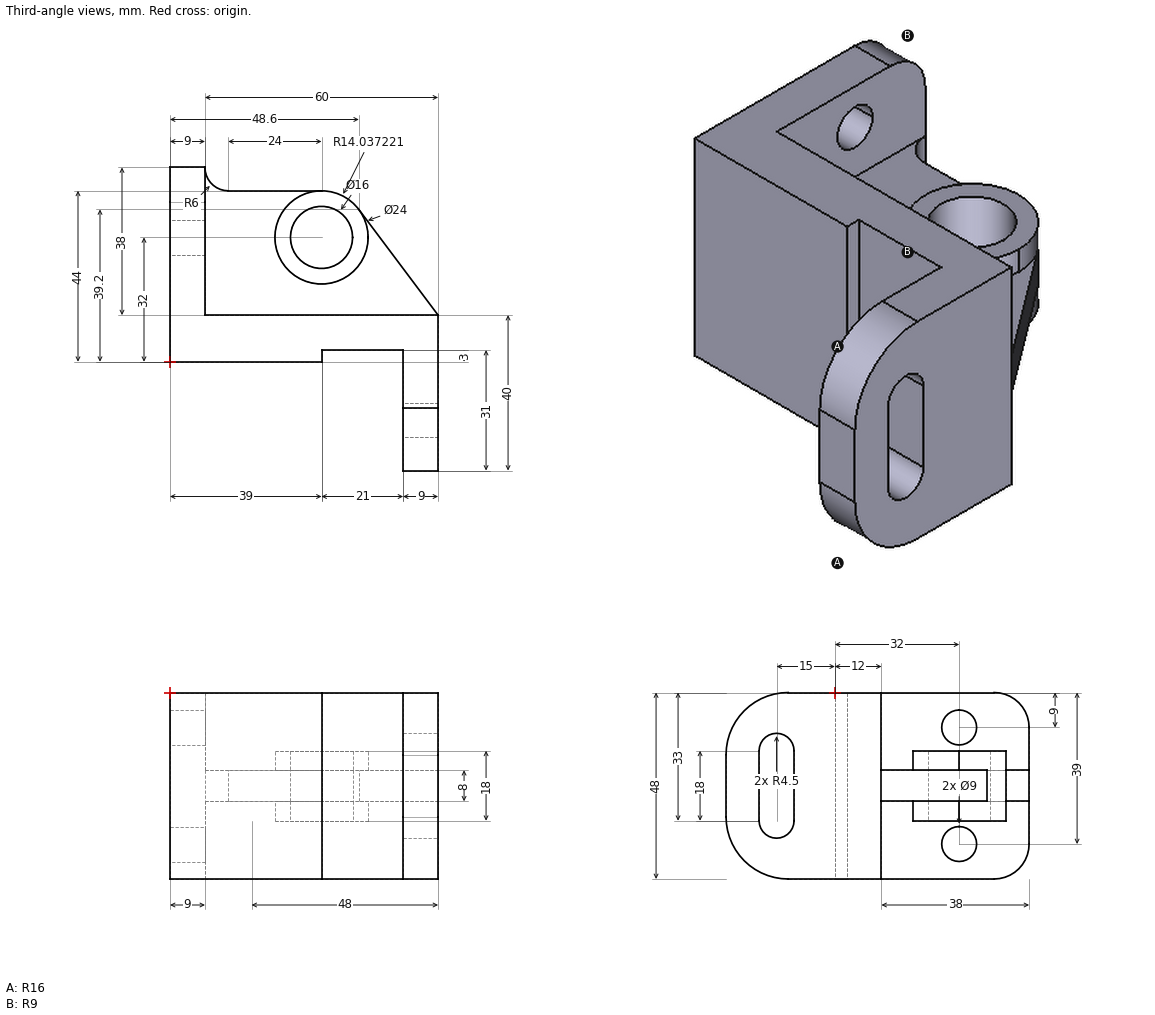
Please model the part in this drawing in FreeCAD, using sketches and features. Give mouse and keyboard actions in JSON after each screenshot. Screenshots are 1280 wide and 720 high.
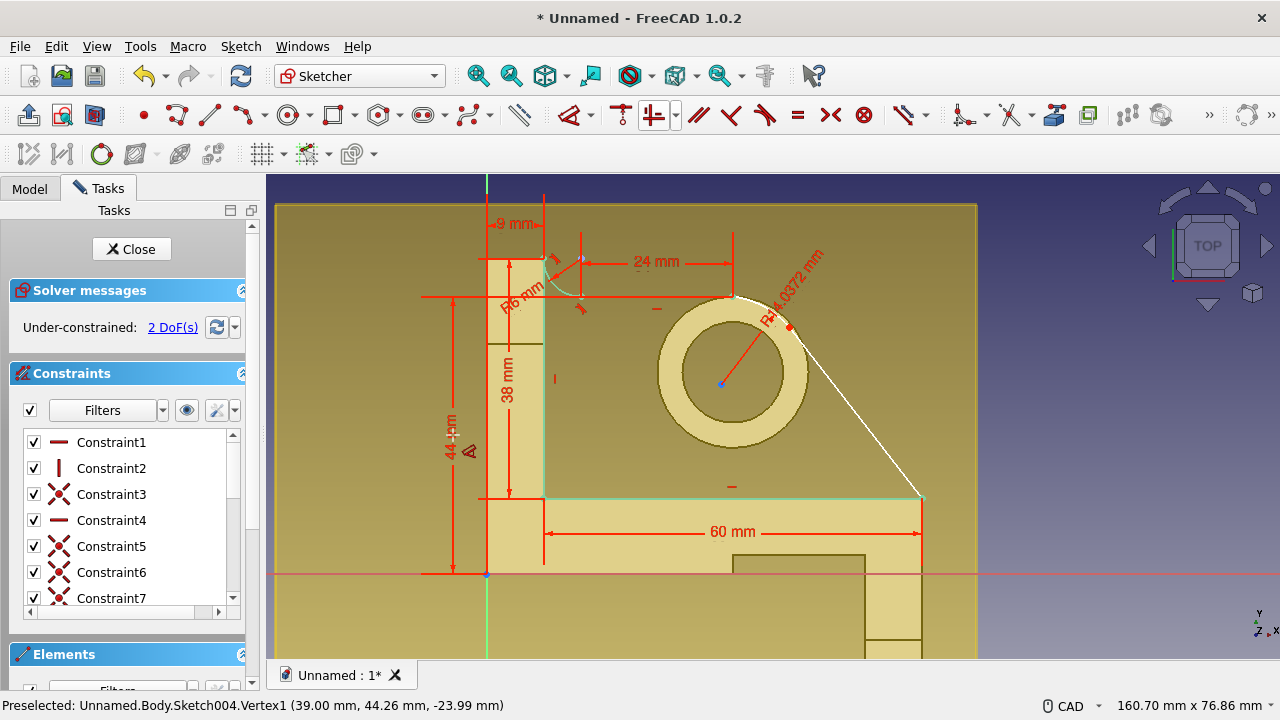
{"action": "left_click", "coordinate": [790, 328]}
{"action": "left_click", "coordinate": [638, 608]}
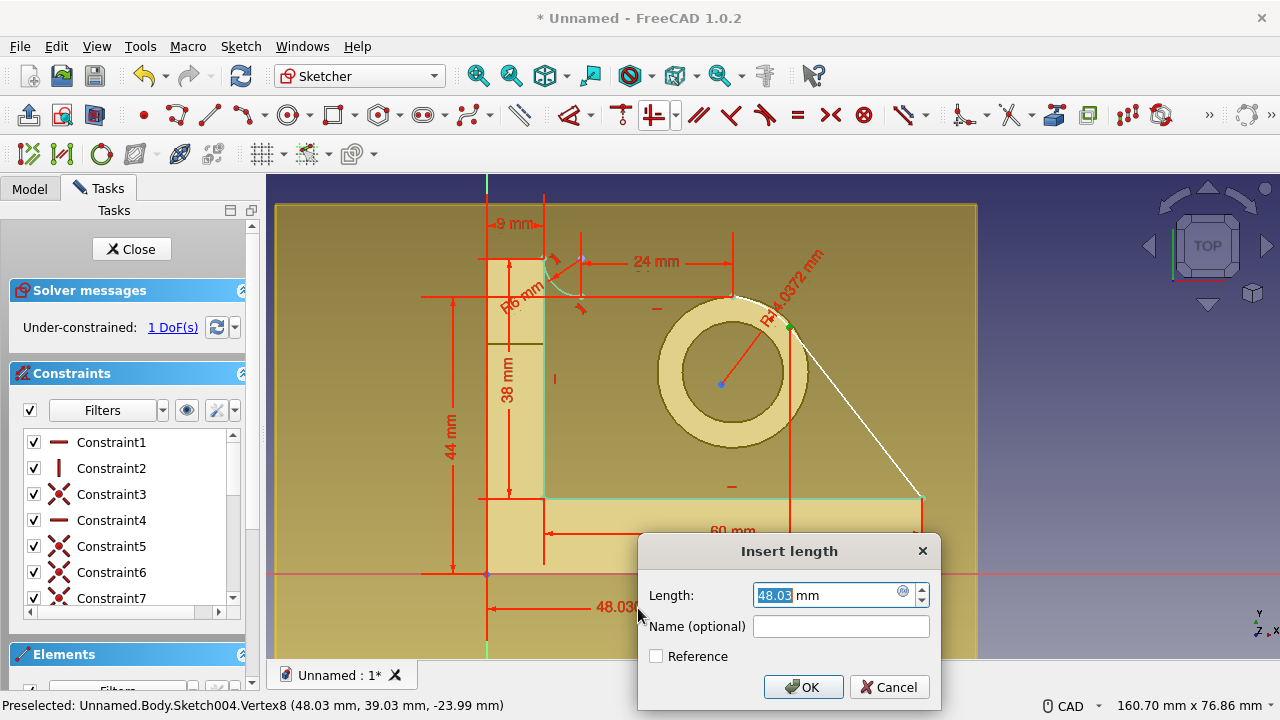
{"action": "type", "text": "48.6"}
{"action": "key", "text": "Return"}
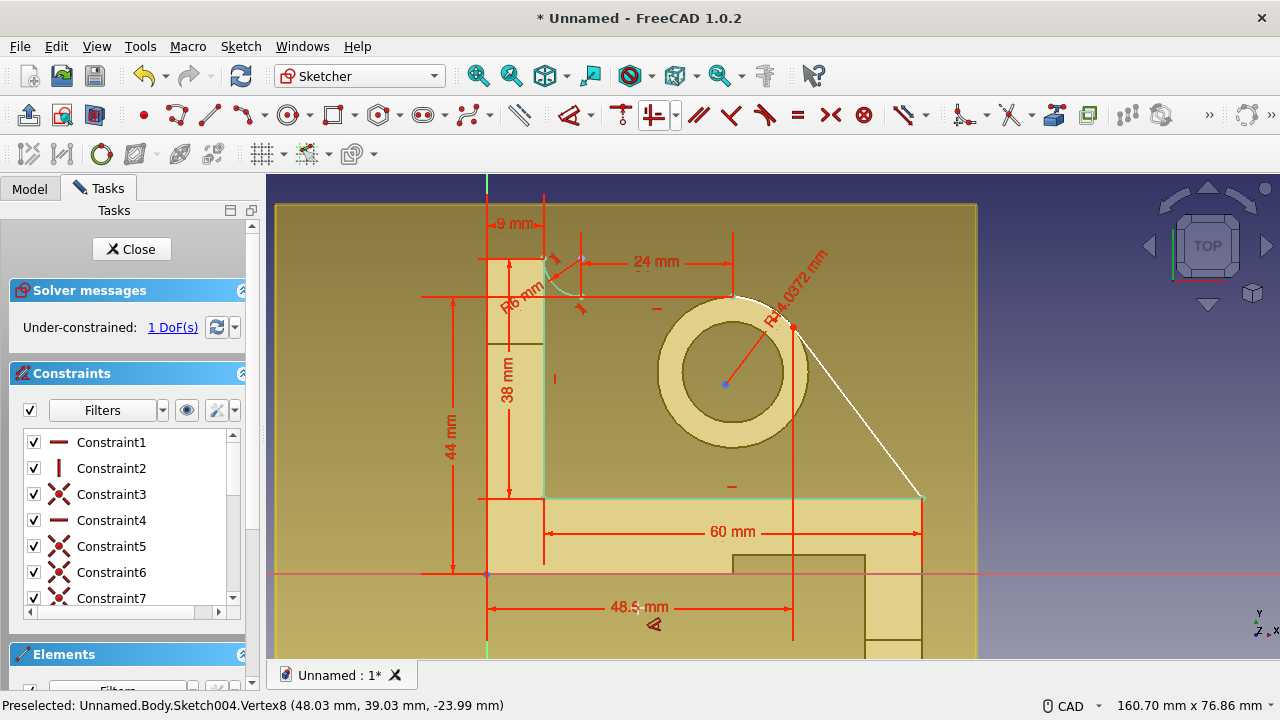
{"action": "left_click", "coordinate": [793, 328]}
{"action": "left_click", "coordinate": [453, 508]}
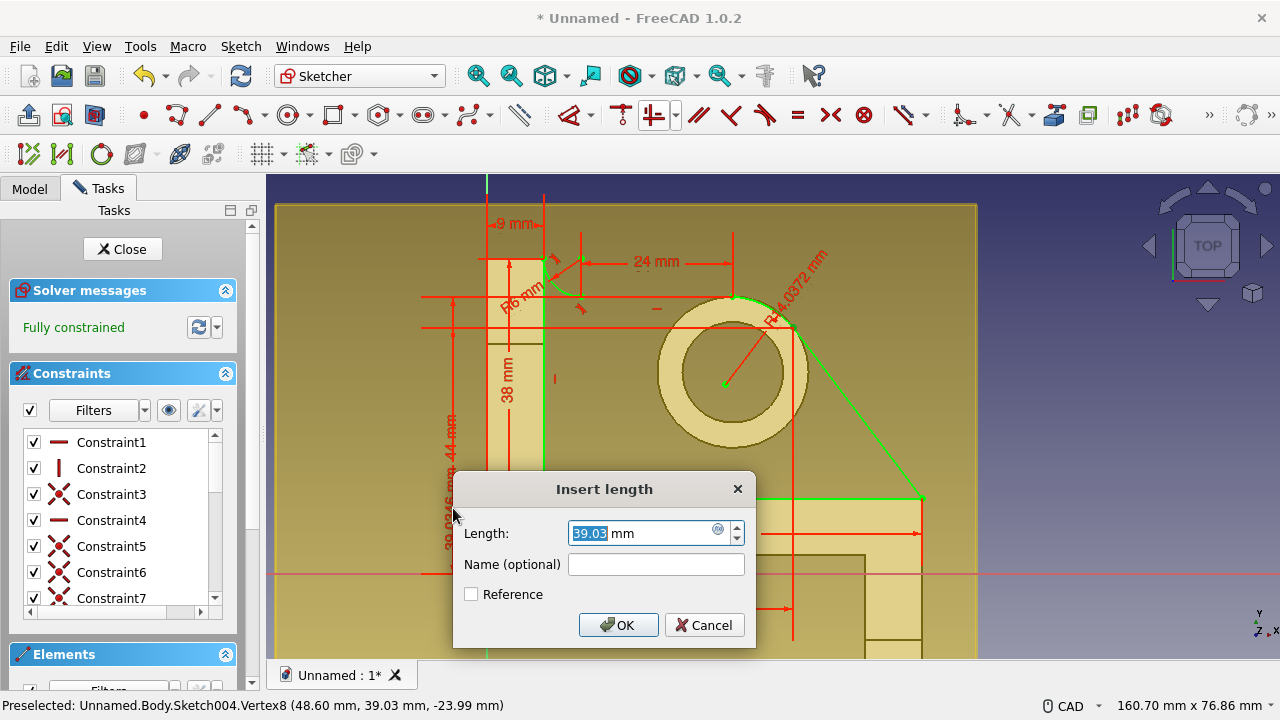
{"action": "type", "text": "39.2"}
{"action": "key", "text": "Return"}
{"action": "key", "text": "Escape"}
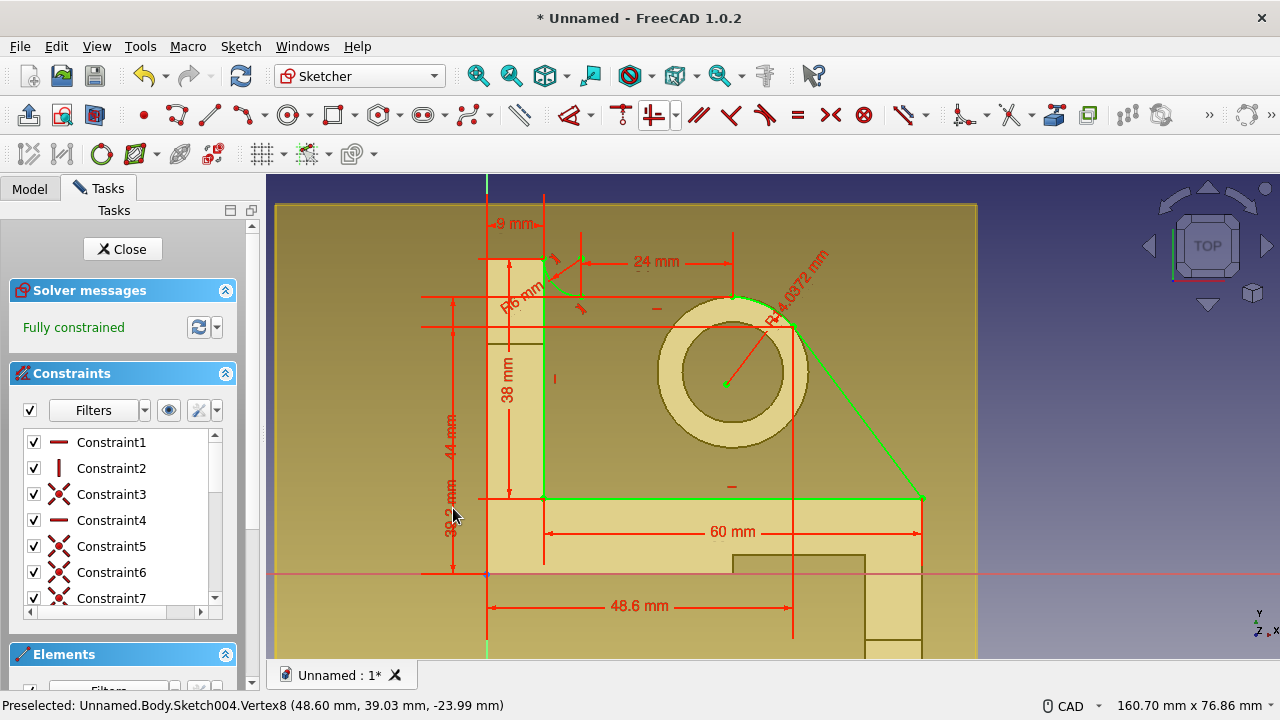
{"action": "left_click", "coordinate": [123, 249]}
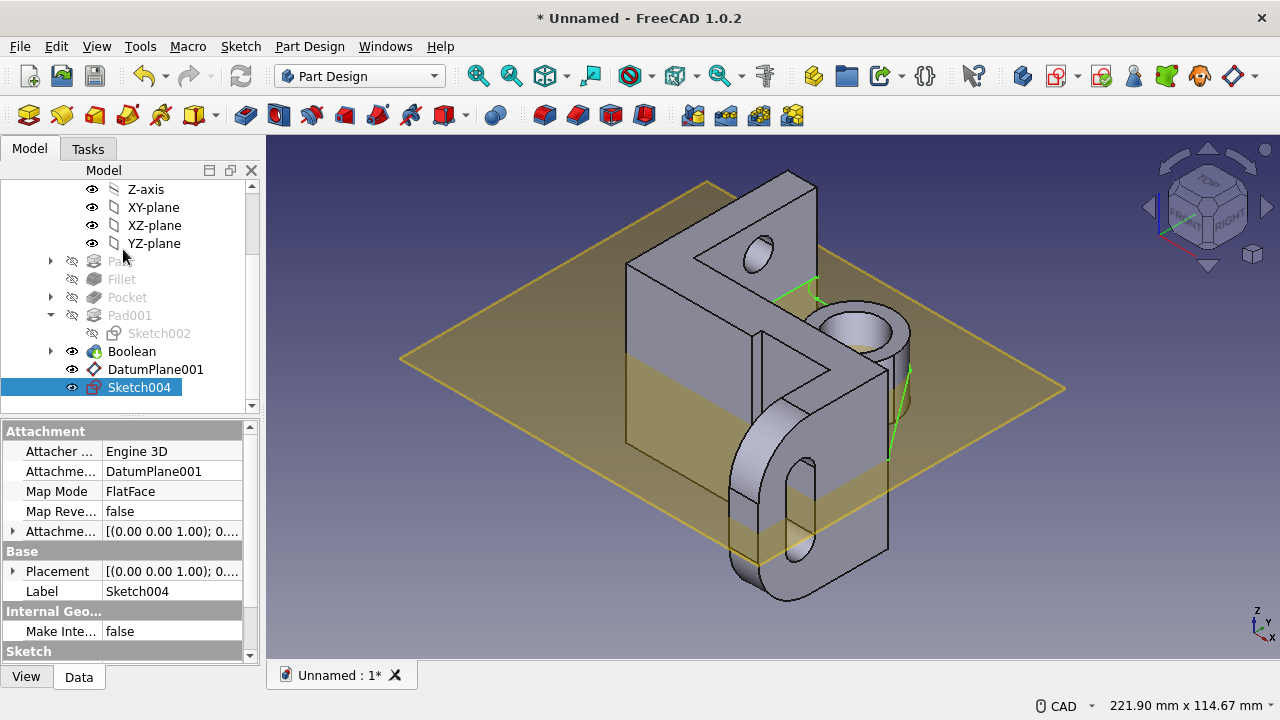
{"action": "left_click", "coordinate": [29, 116]}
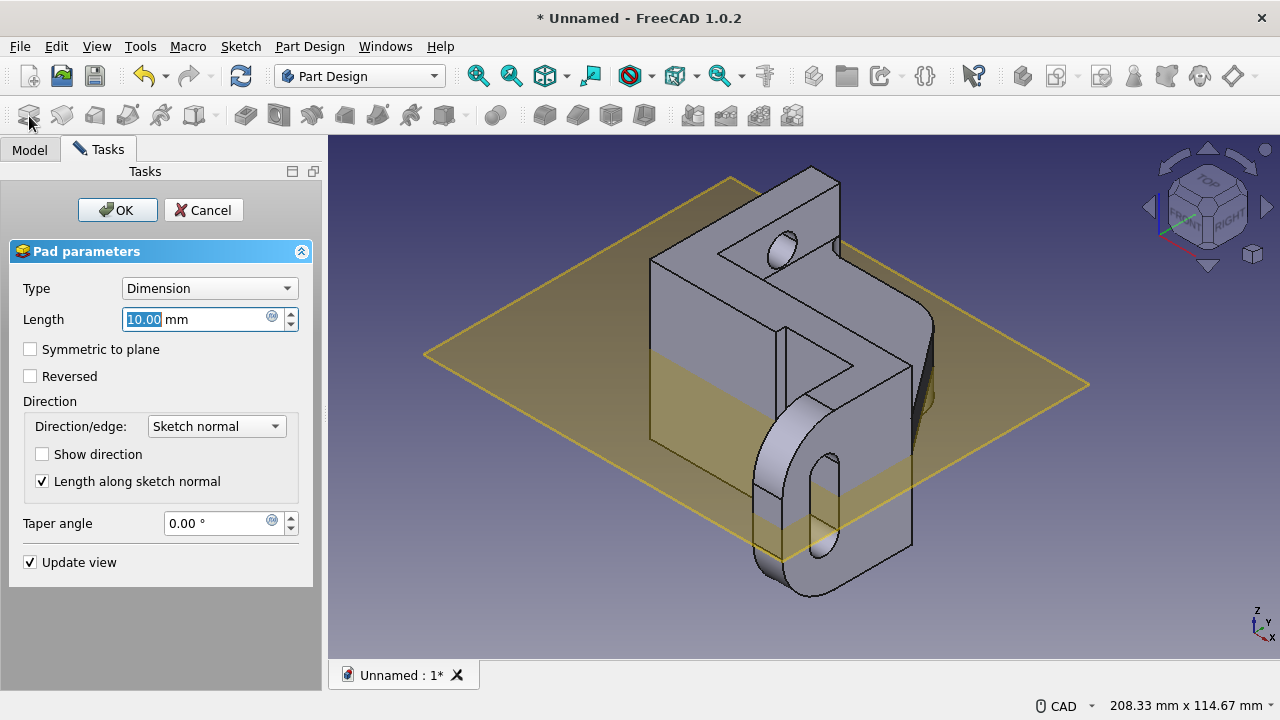
{"action": "type", "text": "8"}
{"action": "key", "text": "Tab"}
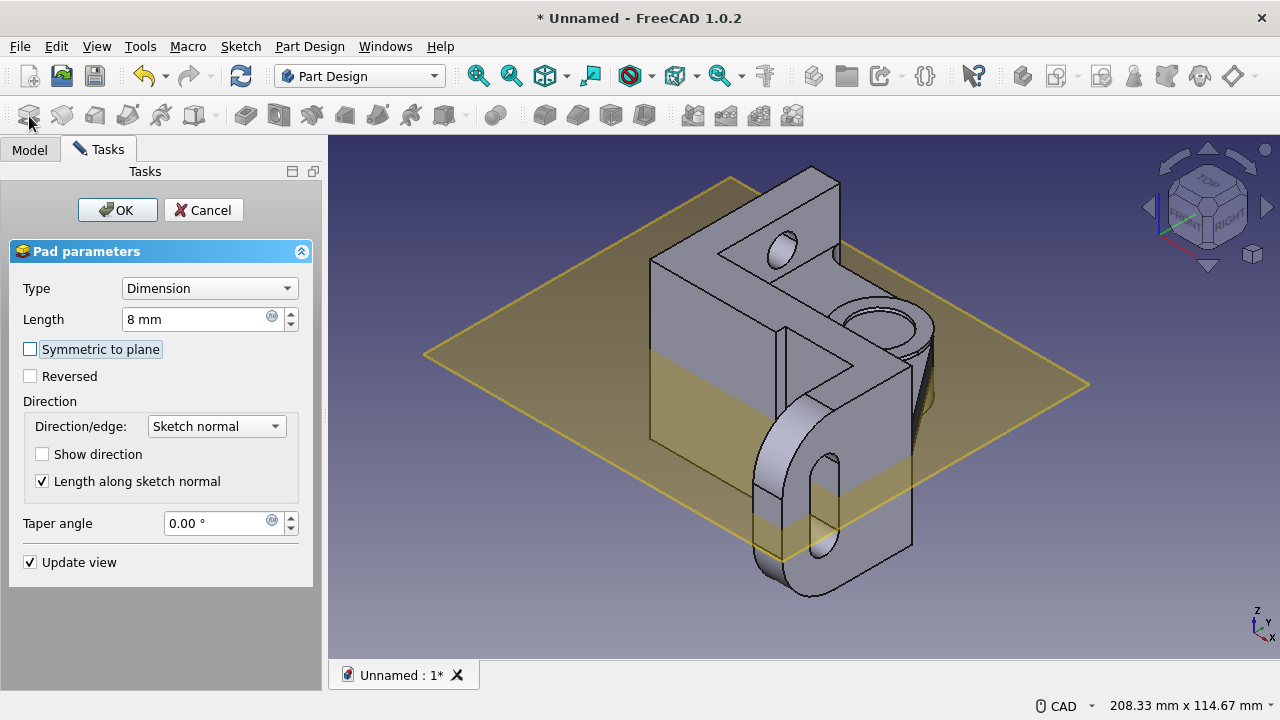
{"action": "left_click", "coordinate": [31, 349]}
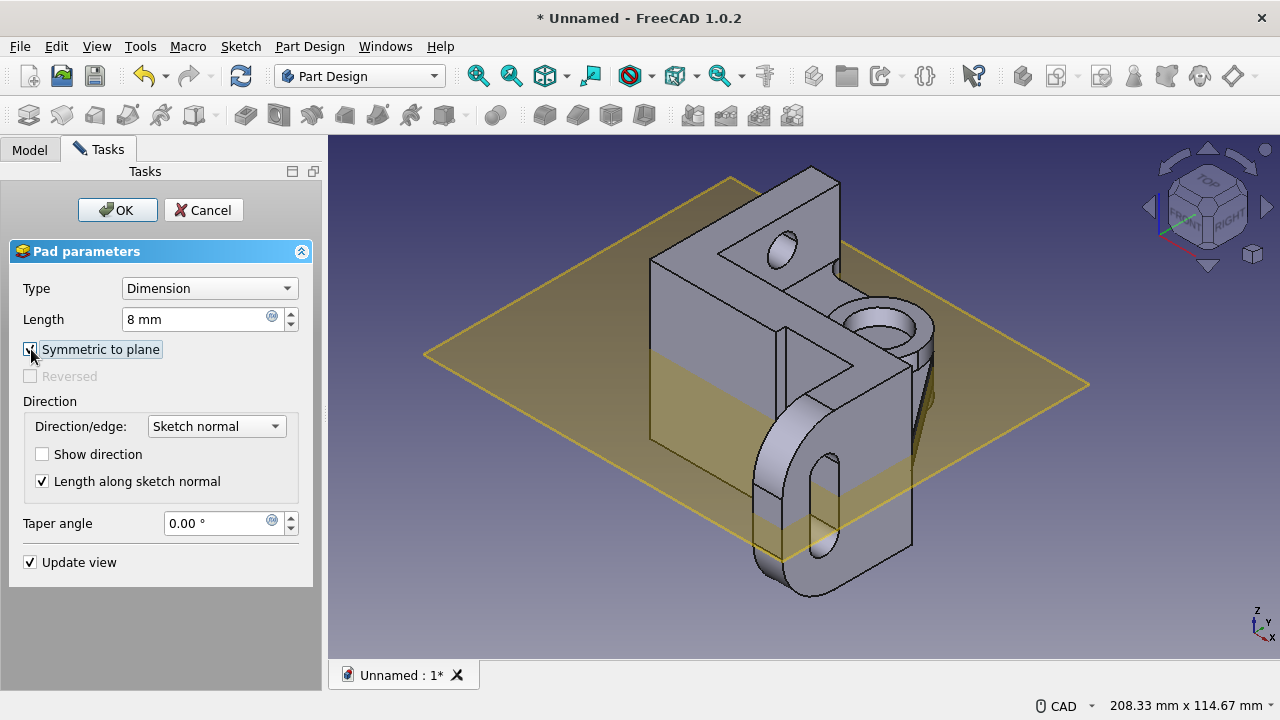
{"action": "left_click", "coordinate": [118, 210]}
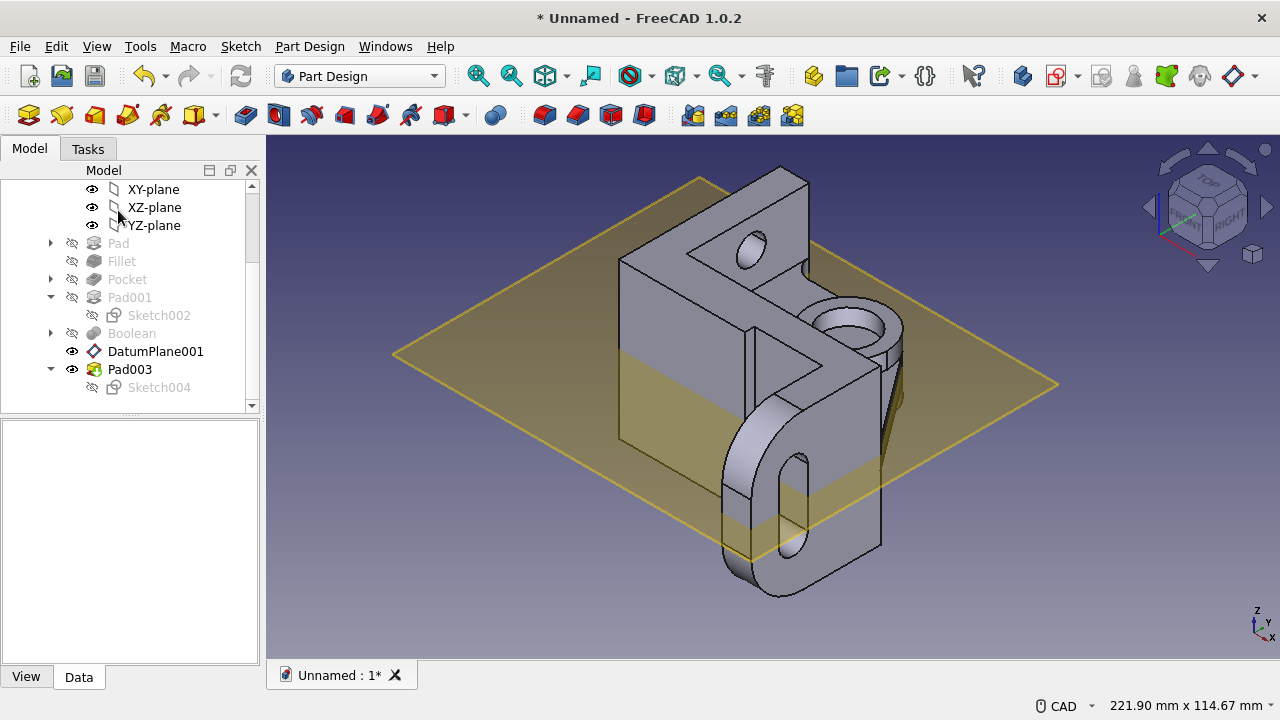
{"action": "left_click", "coordinate": [117, 351]}
{"action": "key", "text": "space"}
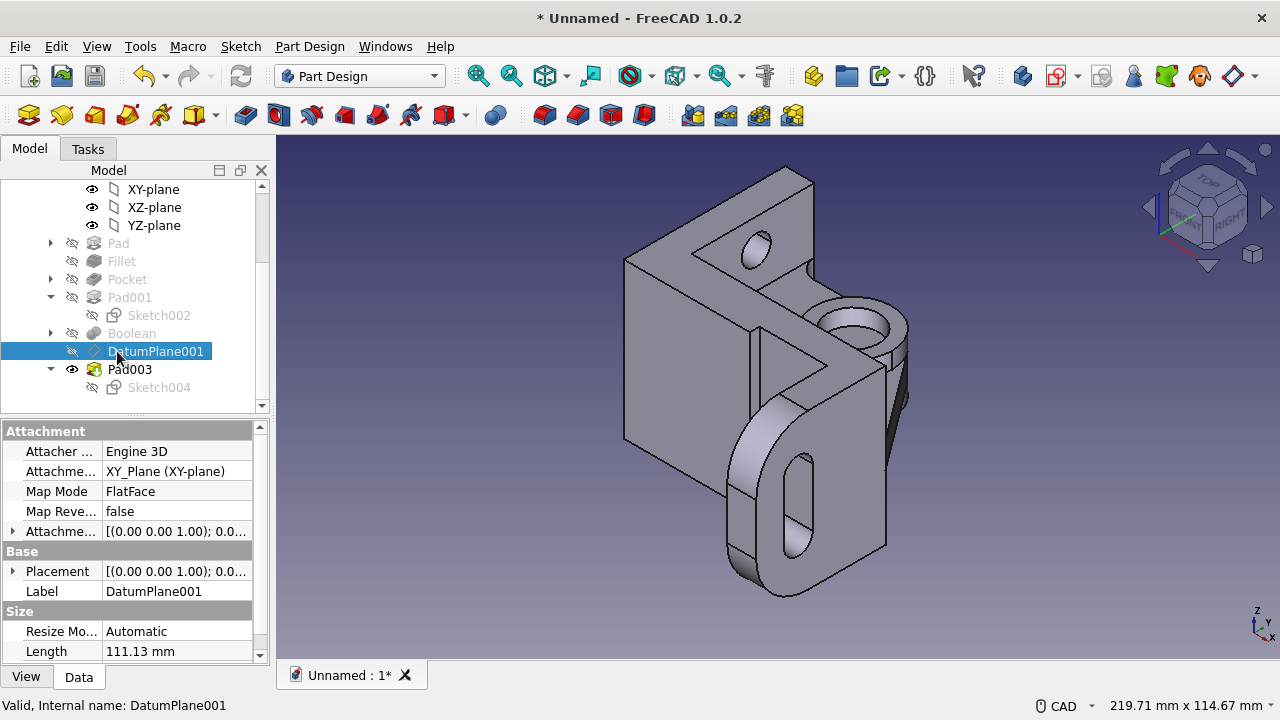
{"action": "left_click", "coordinate": [784, 290]}